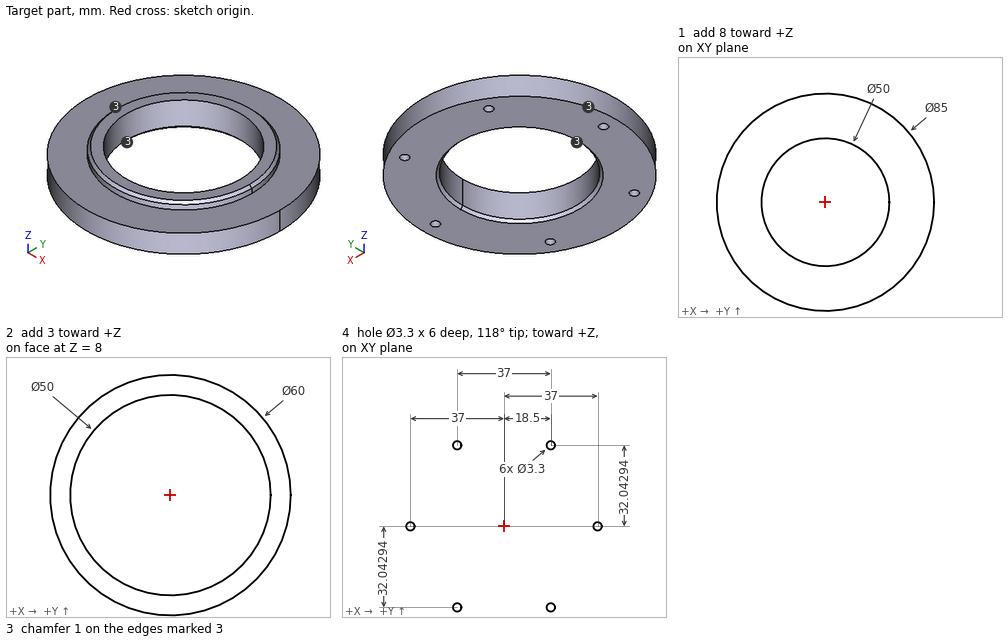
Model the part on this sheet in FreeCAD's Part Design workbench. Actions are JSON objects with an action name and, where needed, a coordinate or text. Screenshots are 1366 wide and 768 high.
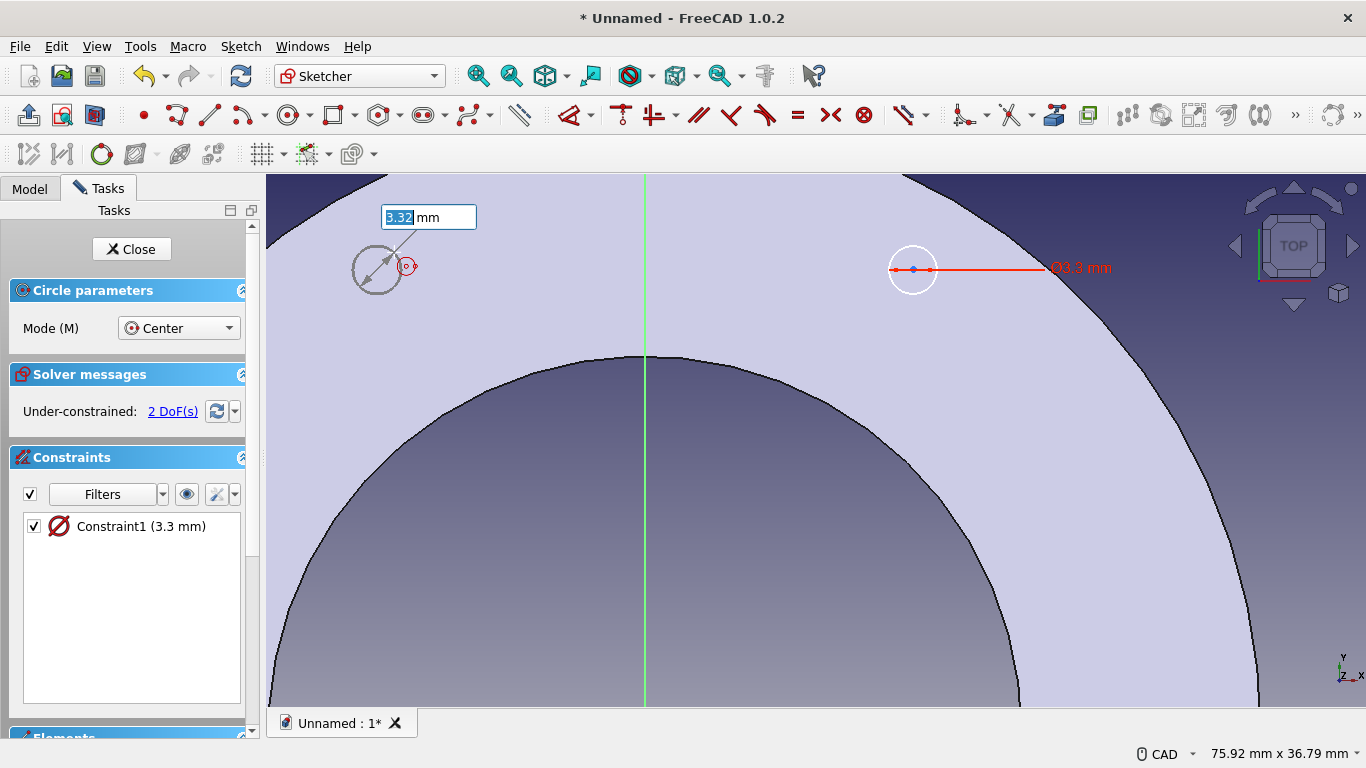
{"action": "type", "text": "3.3"}
{"action": "key", "text": "Return"}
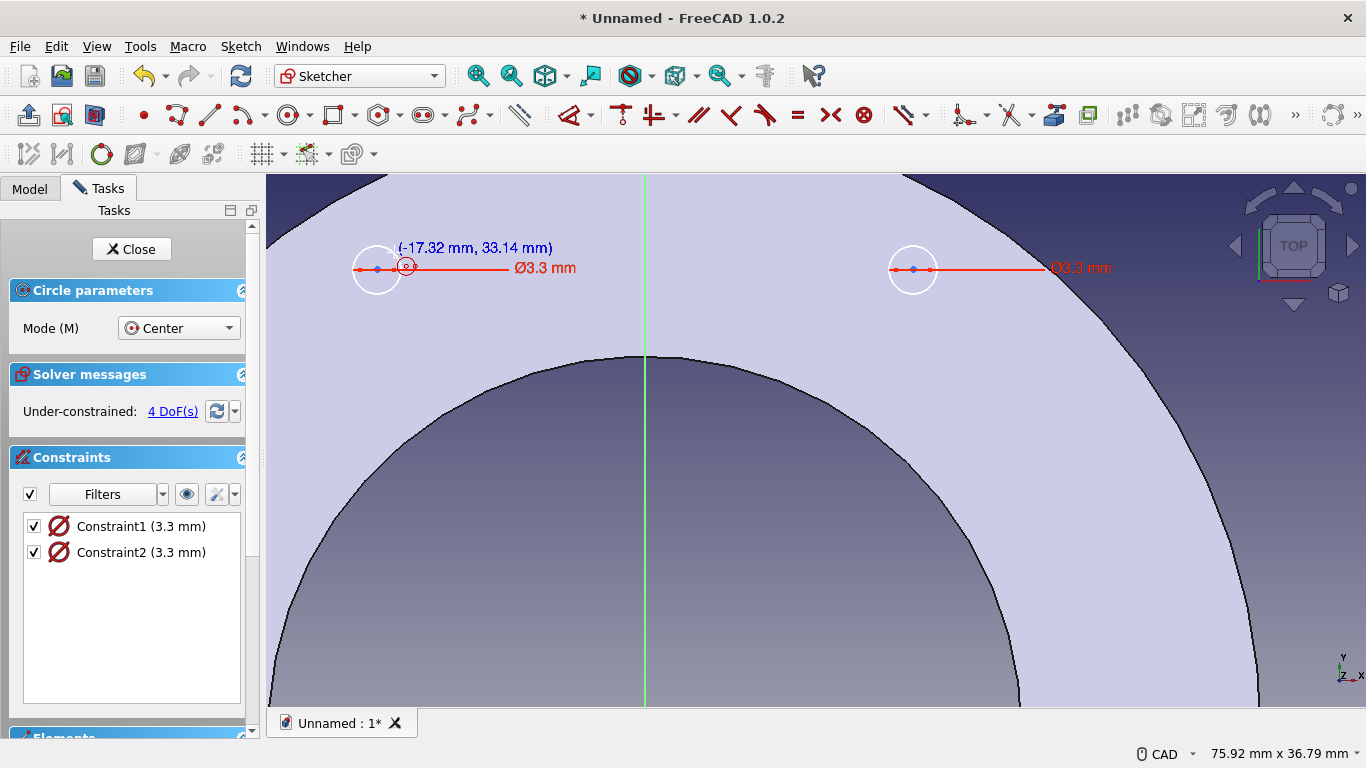
{"action": "scroll", "coordinate": [807, 270], "scroll_direction": "down", "scroll_amount": 5}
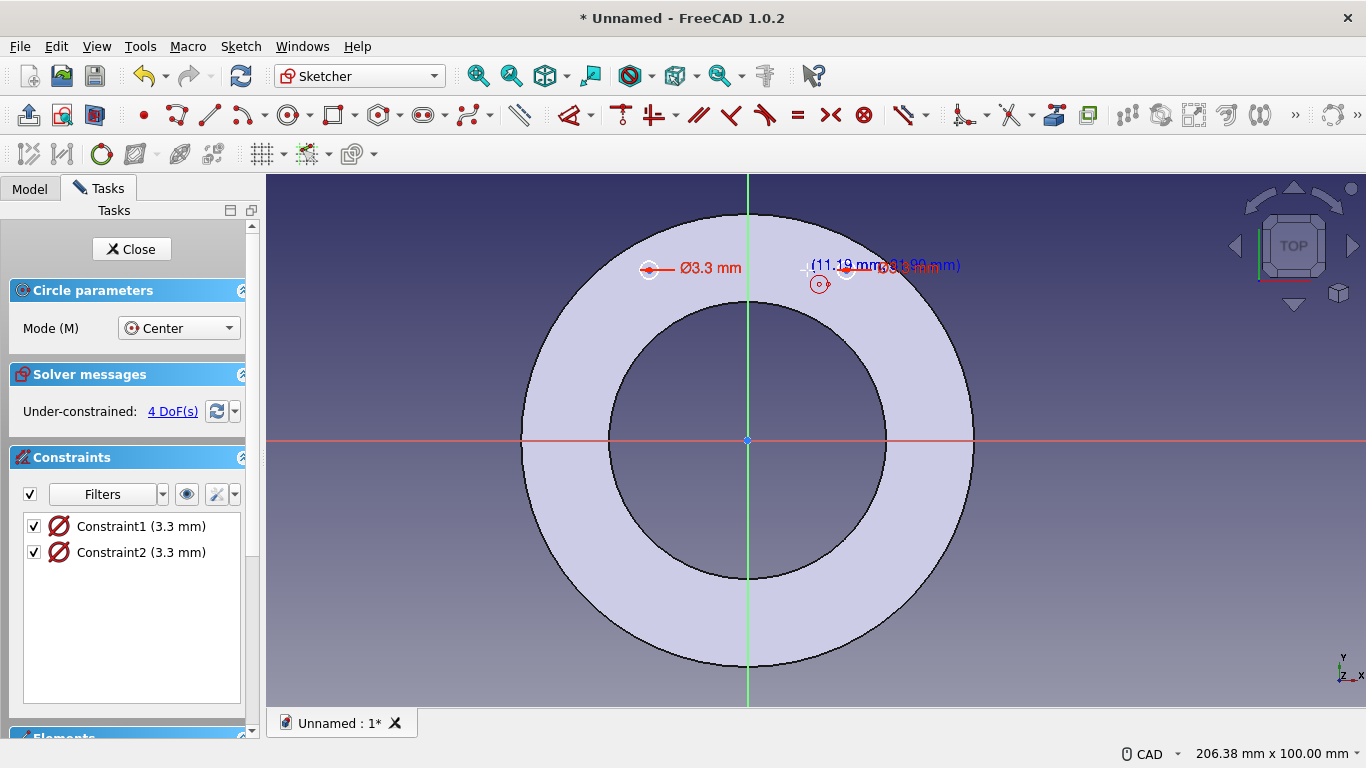
{"action": "scroll", "coordinate": [550, 440], "scroll_direction": "up", "scroll_amount": 5}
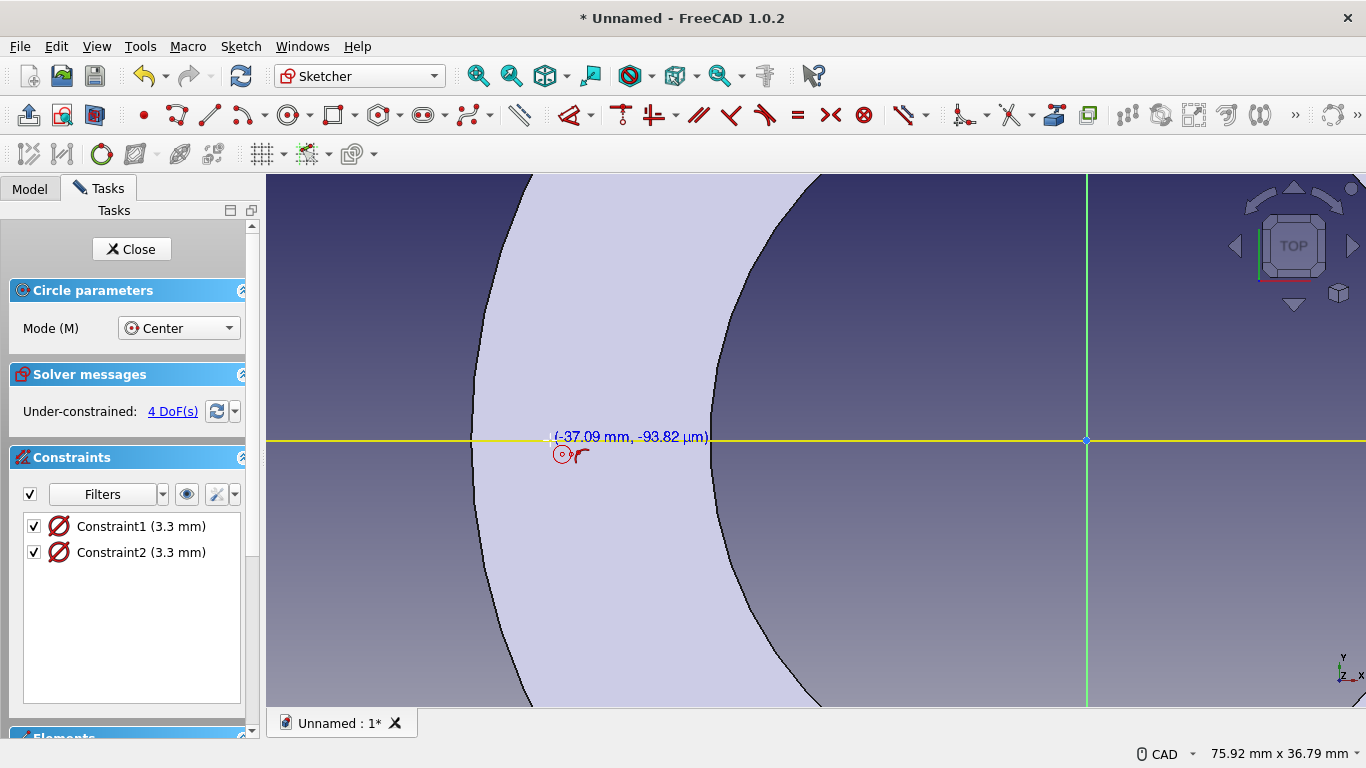
{"action": "left_click", "coordinate": [551, 440]}
{"action": "mouse_move", "coordinate": [568, 424]}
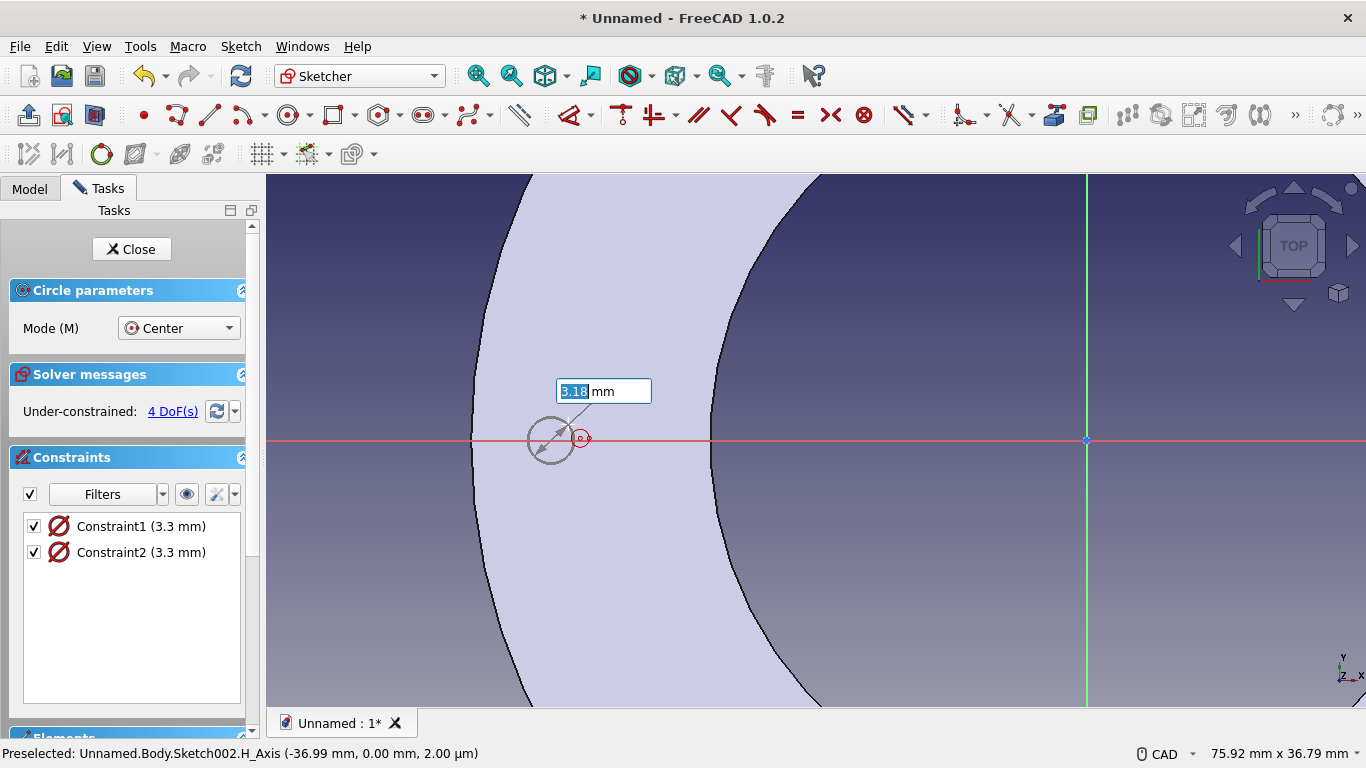
{"action": "type", "text": "3.3"}
{"action": "key", "text": "Return"}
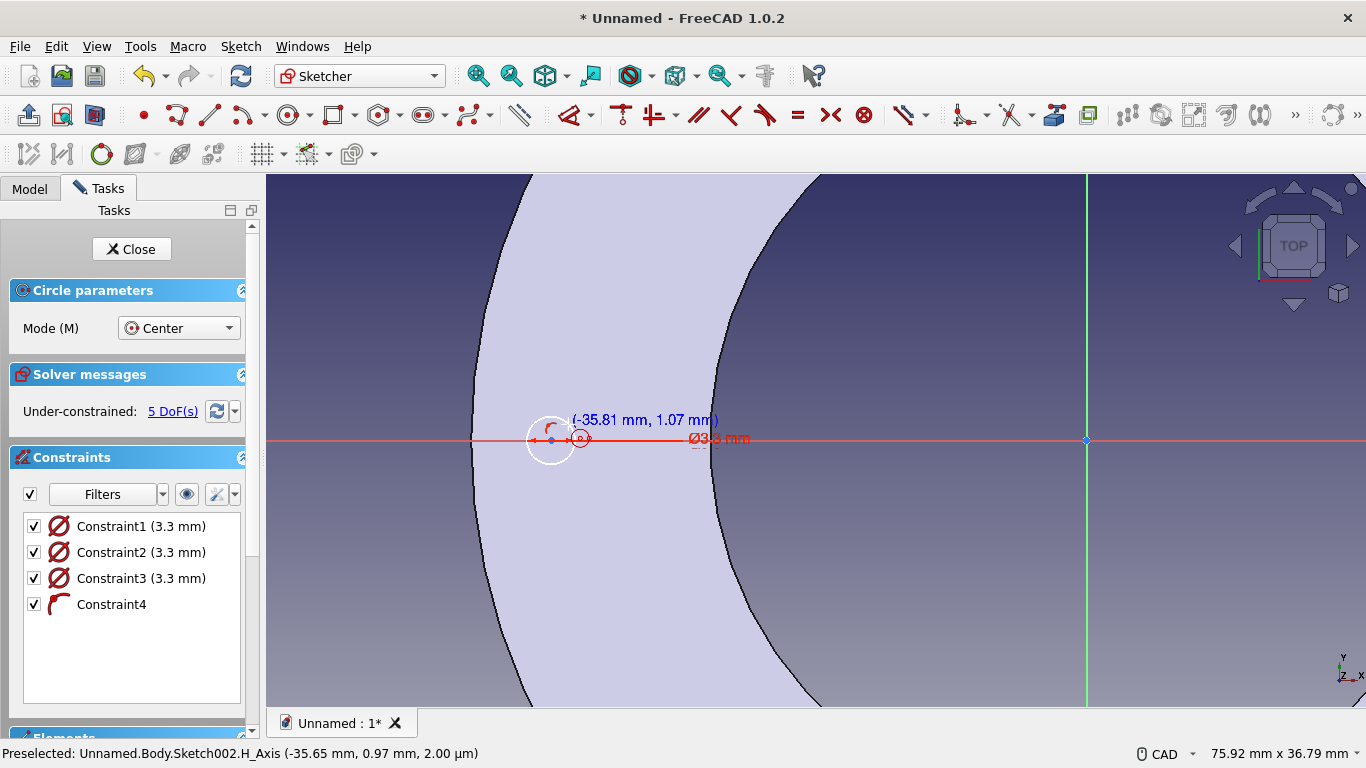
{"action": "scroll", "coordinate": [550, 441], "scroll_direction": "down", "scroll_amount": 5}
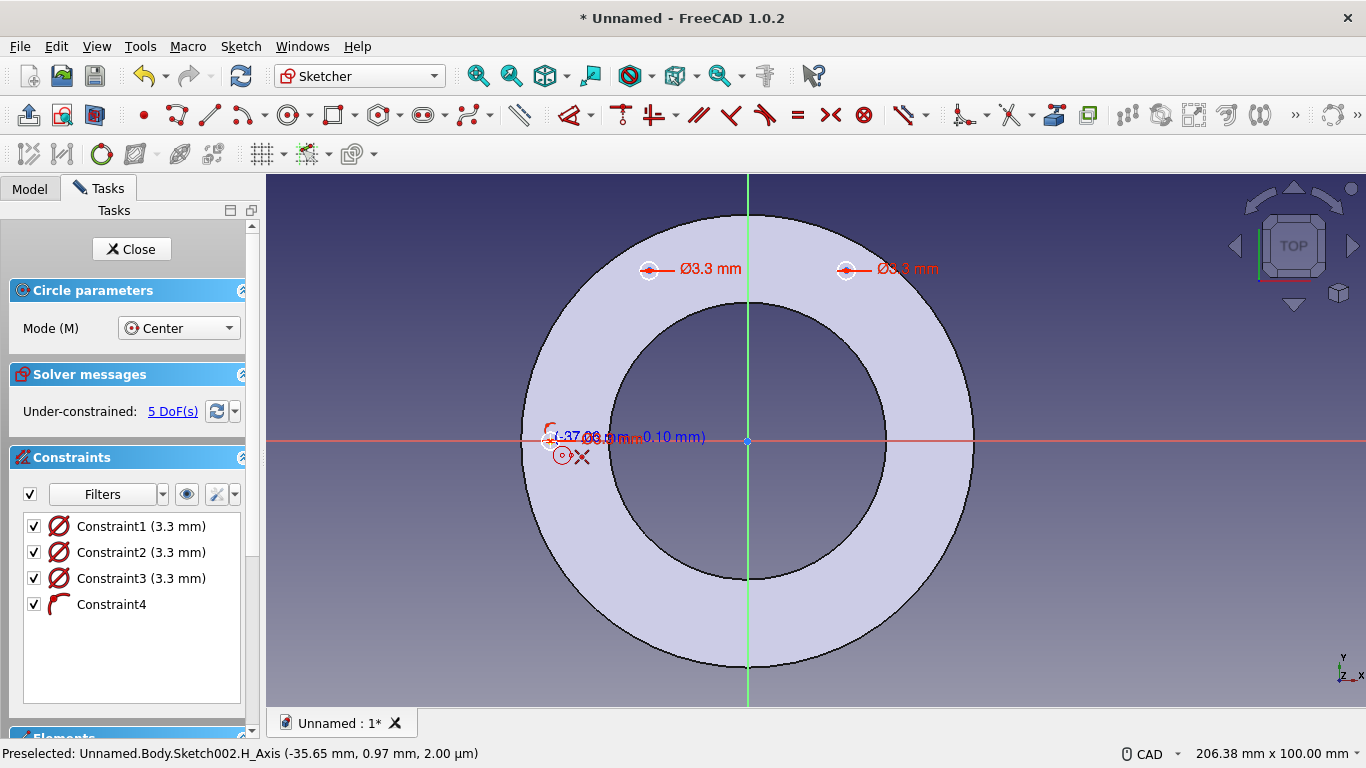
{"action": "scroll", "coordinate": [649, 612], "scroll_direction": "up", "scroll_amount": 5}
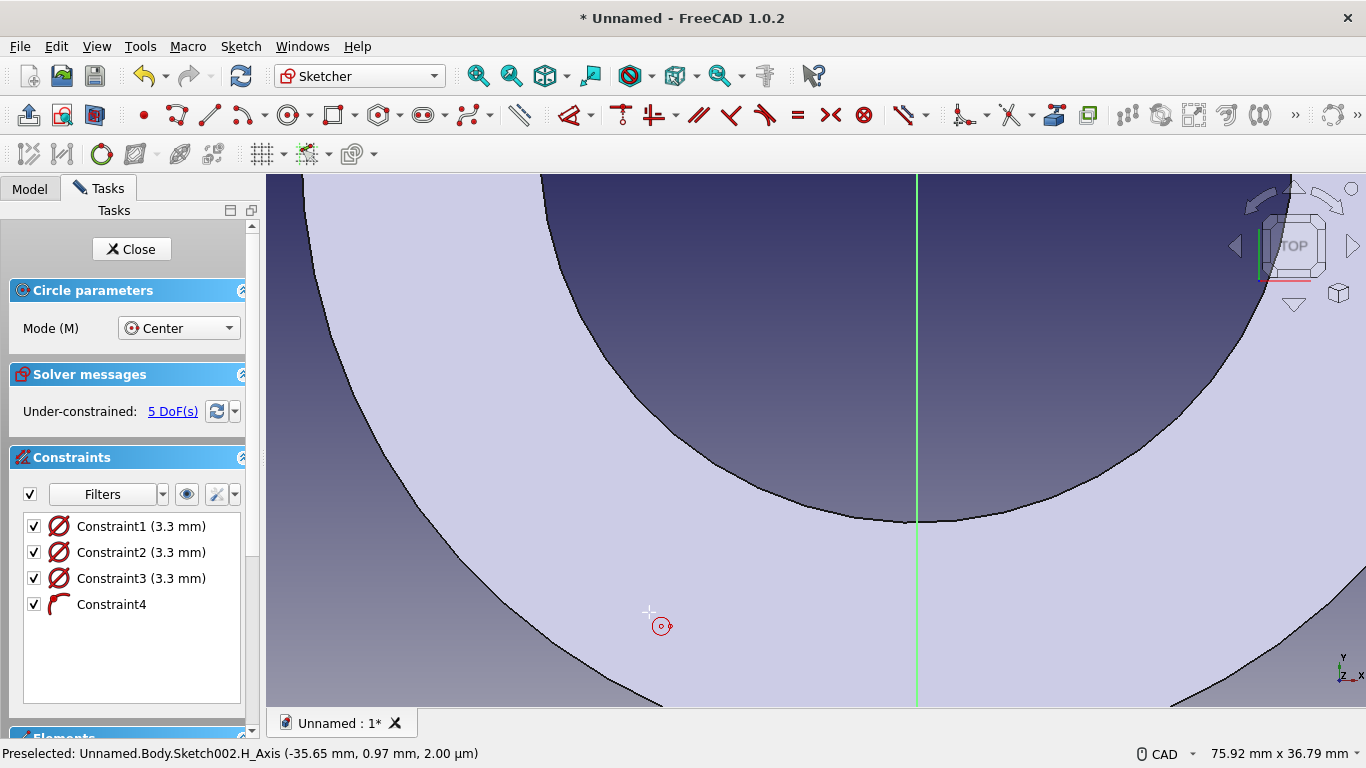
{"action": "left_click", "coordinate": [649, 610]}
{"action": "mouse_move", "coordinate": [665, 593]}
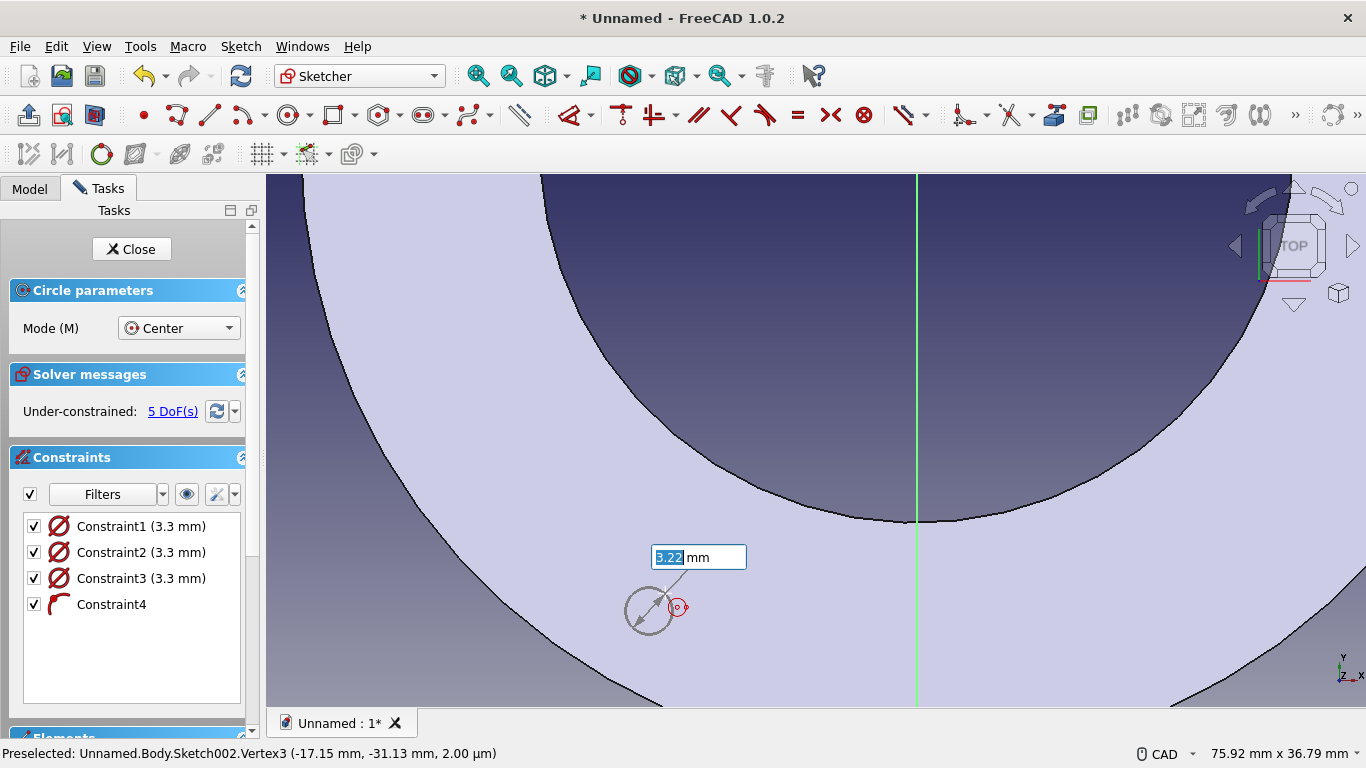
{"action": "type", "text": "3.3"}
{"action": "key", "text": "Return"}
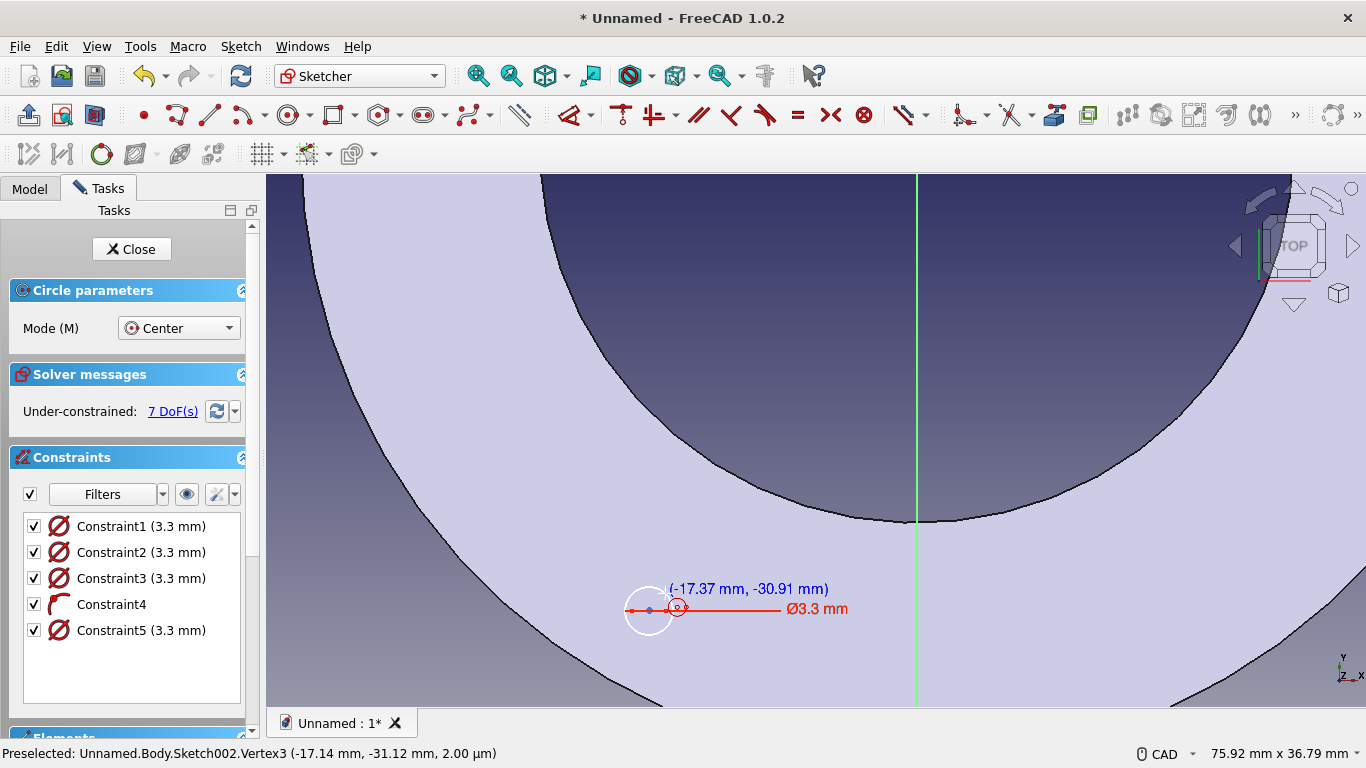
{"action": "left_click", "coordinate": [1185, 610]}